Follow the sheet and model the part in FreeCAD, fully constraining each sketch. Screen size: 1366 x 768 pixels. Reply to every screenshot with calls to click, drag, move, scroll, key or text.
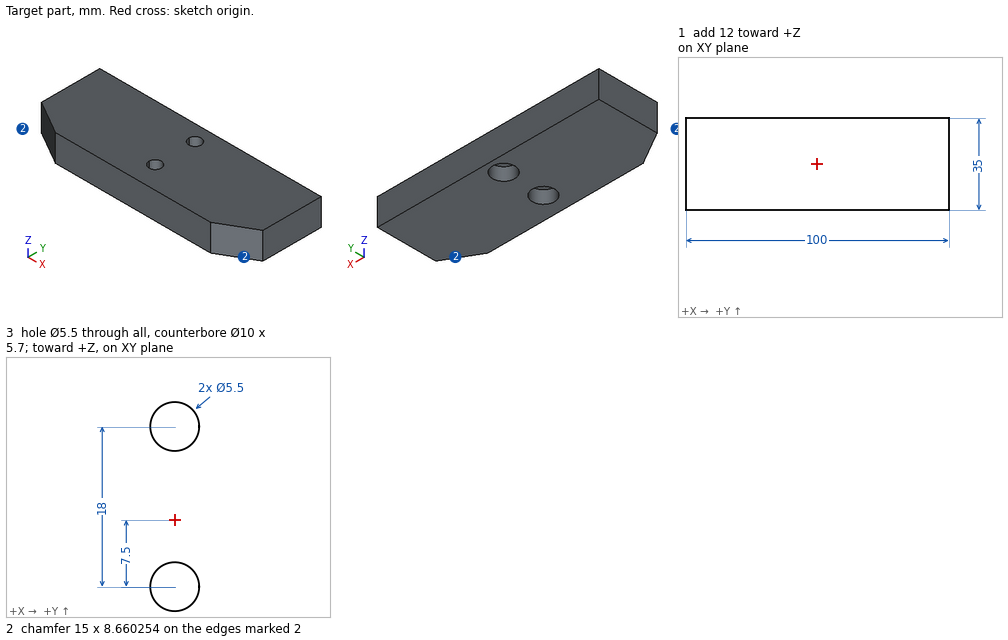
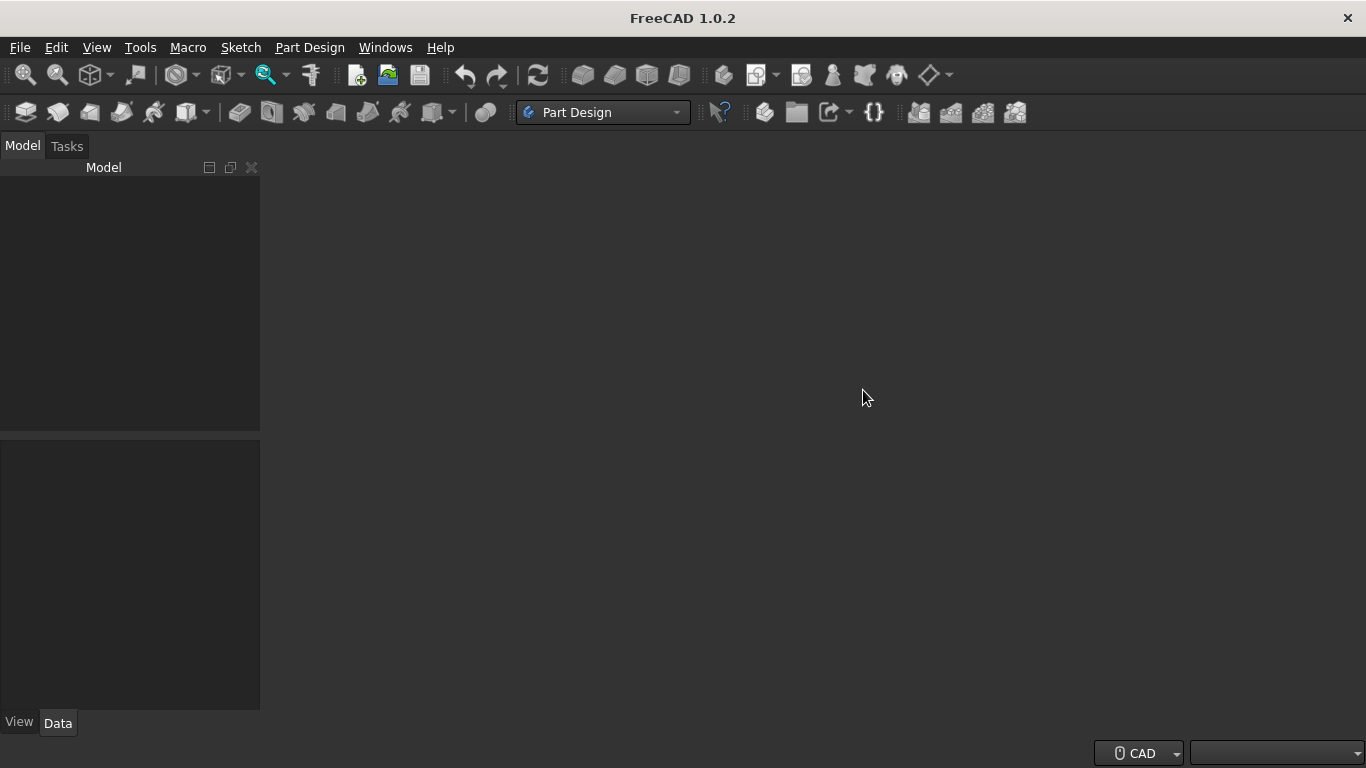
click(356, 76)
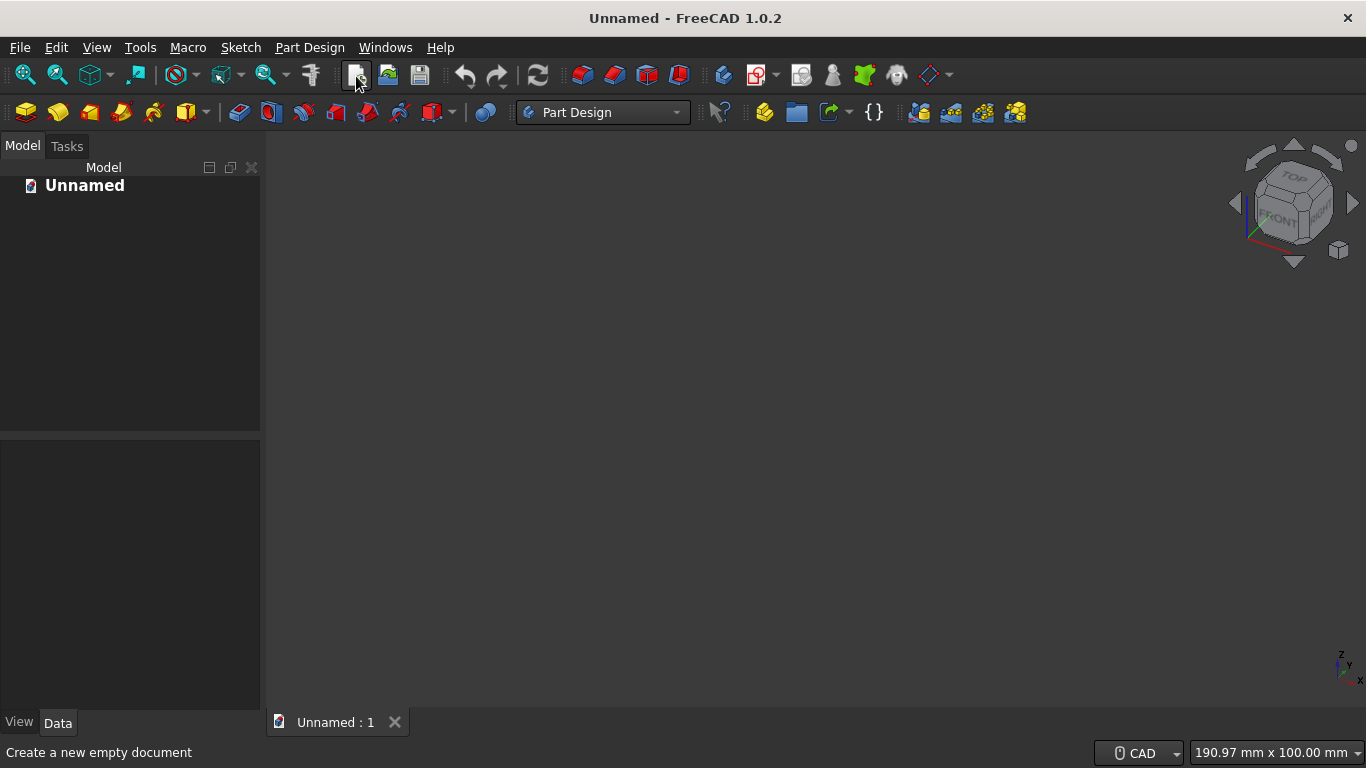
click(756, 76)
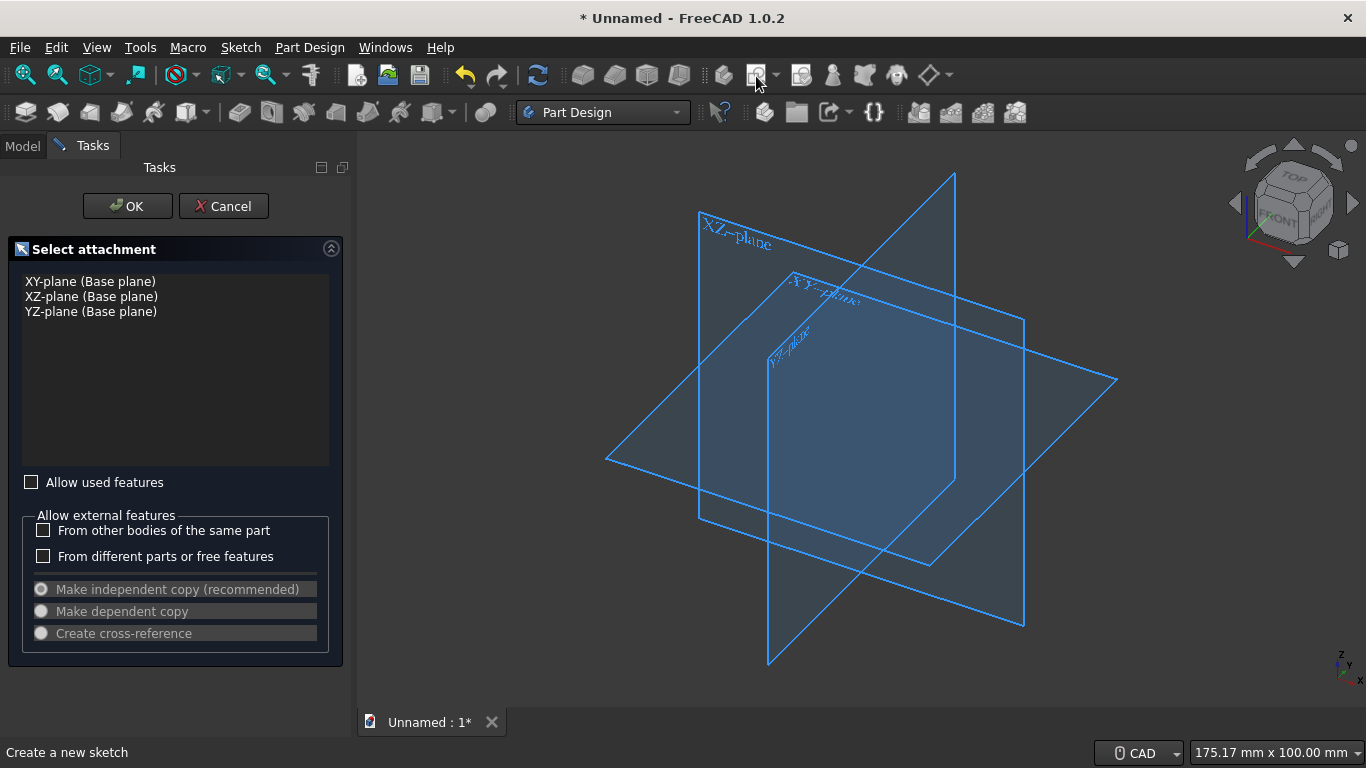
click(82, 282)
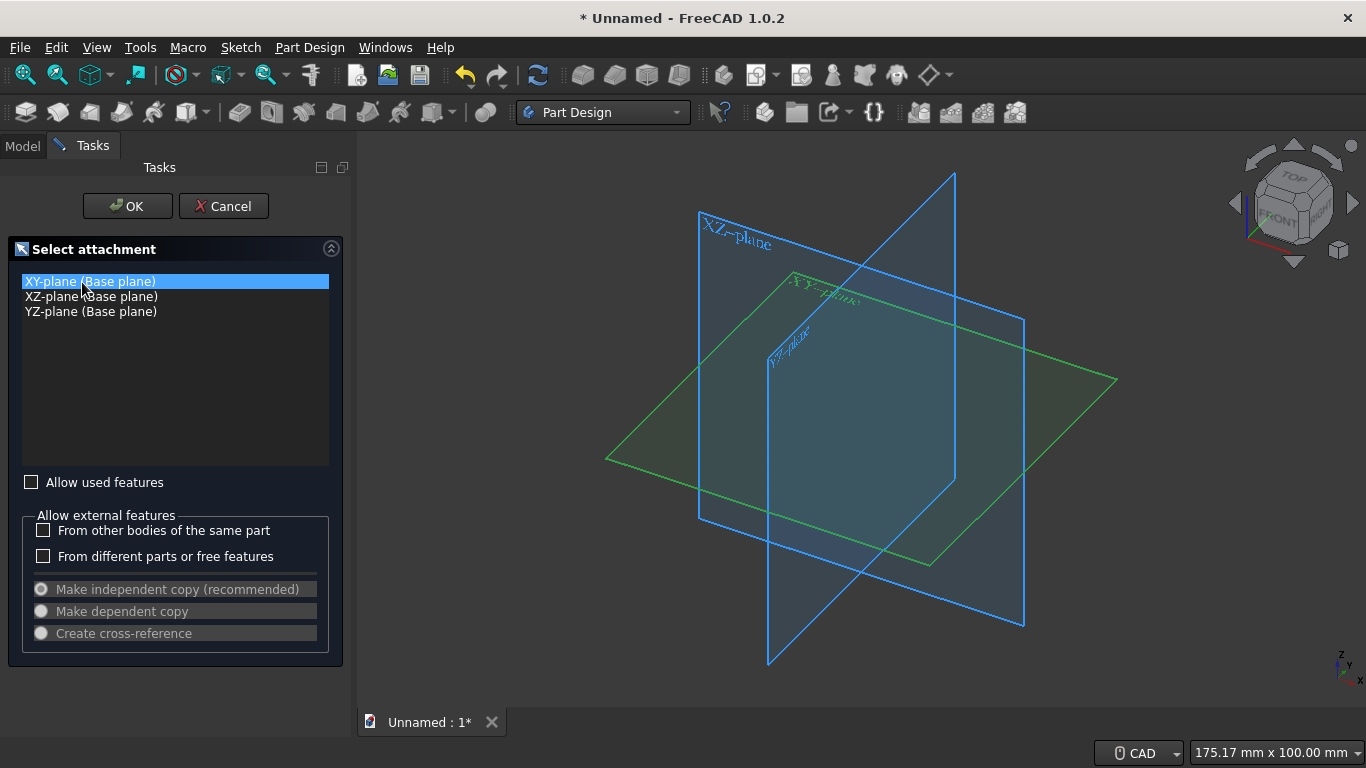
click(128, 206)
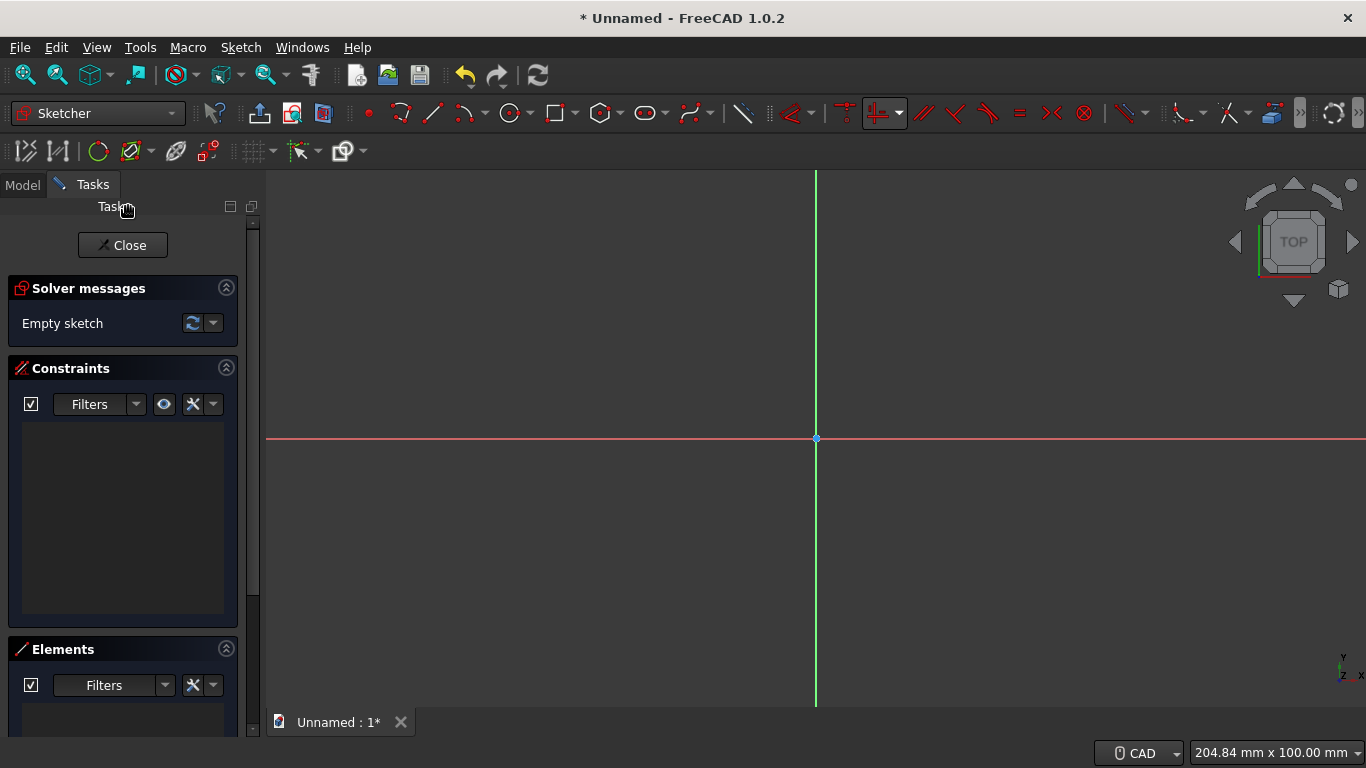
click(578, 114)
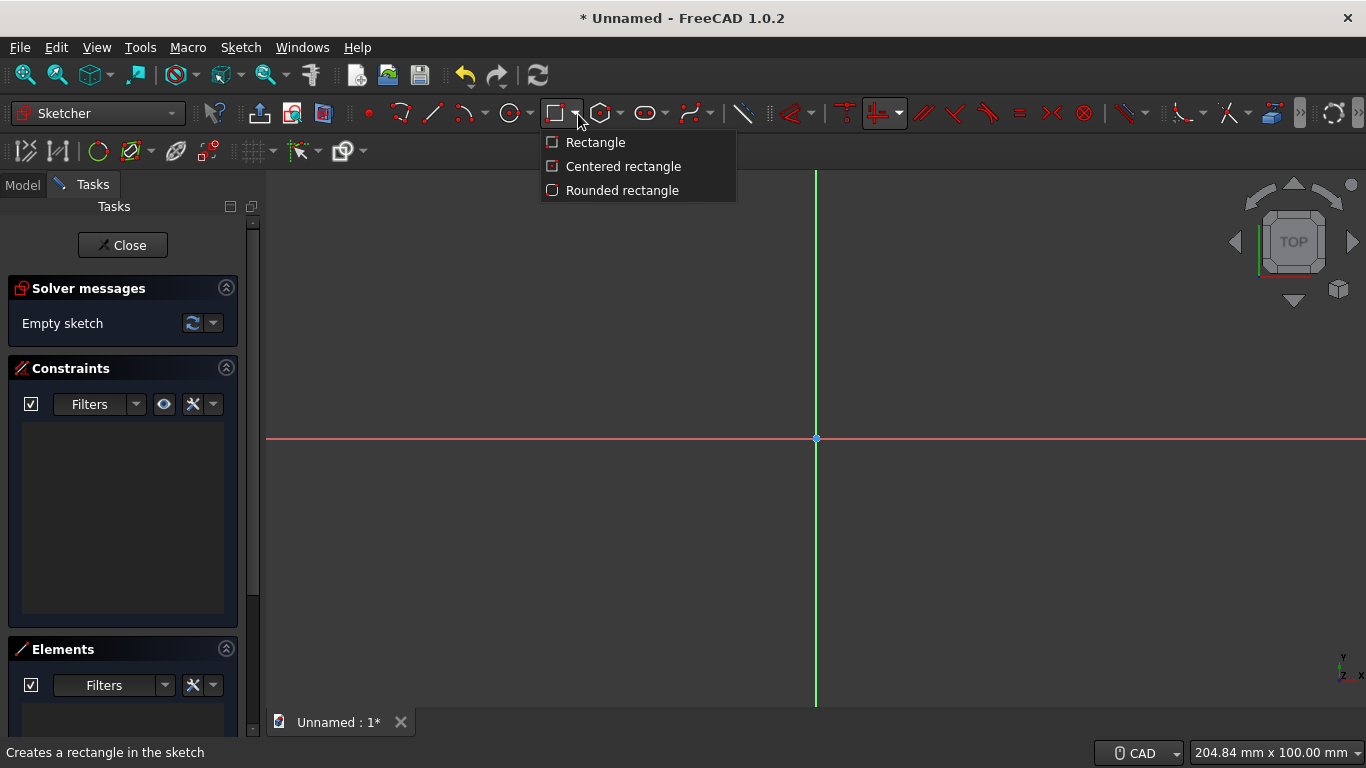
click(638, 166)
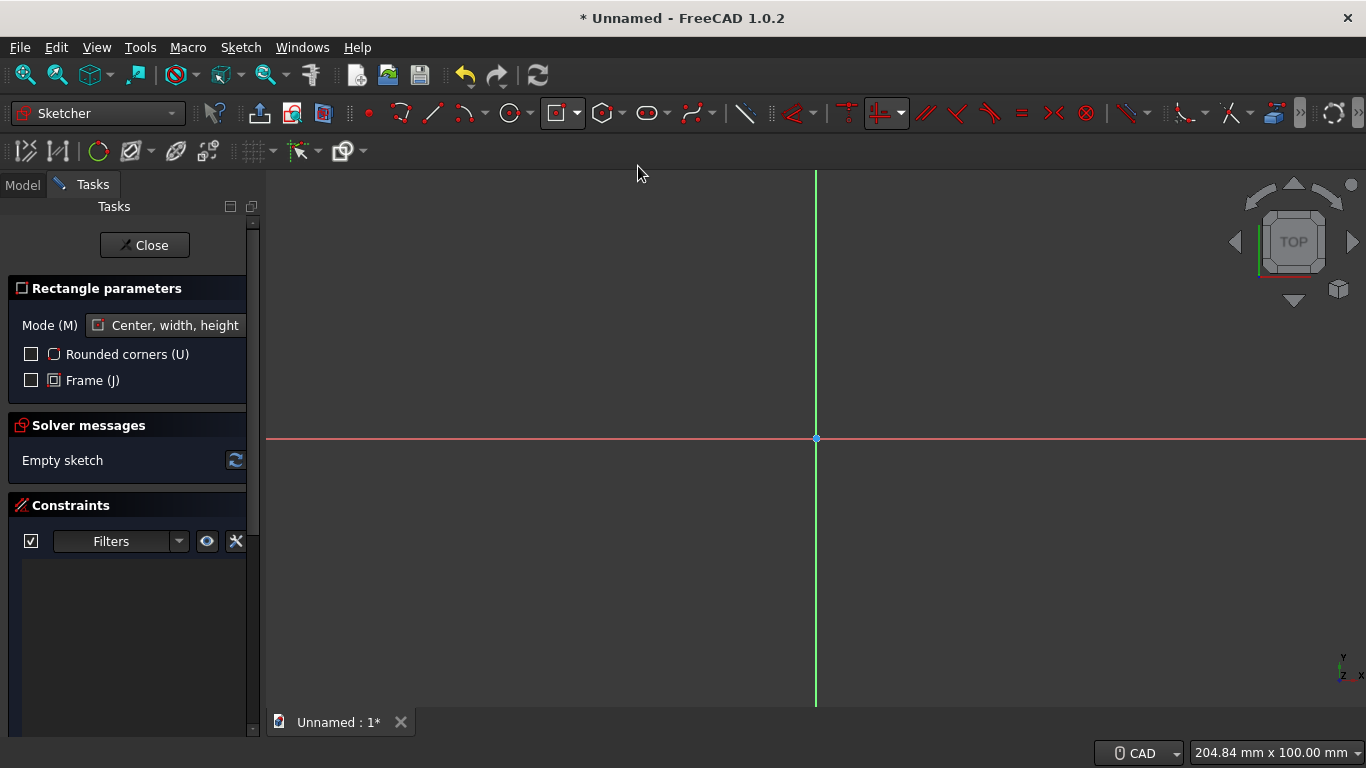
click(816, 438)
move(1084, 345)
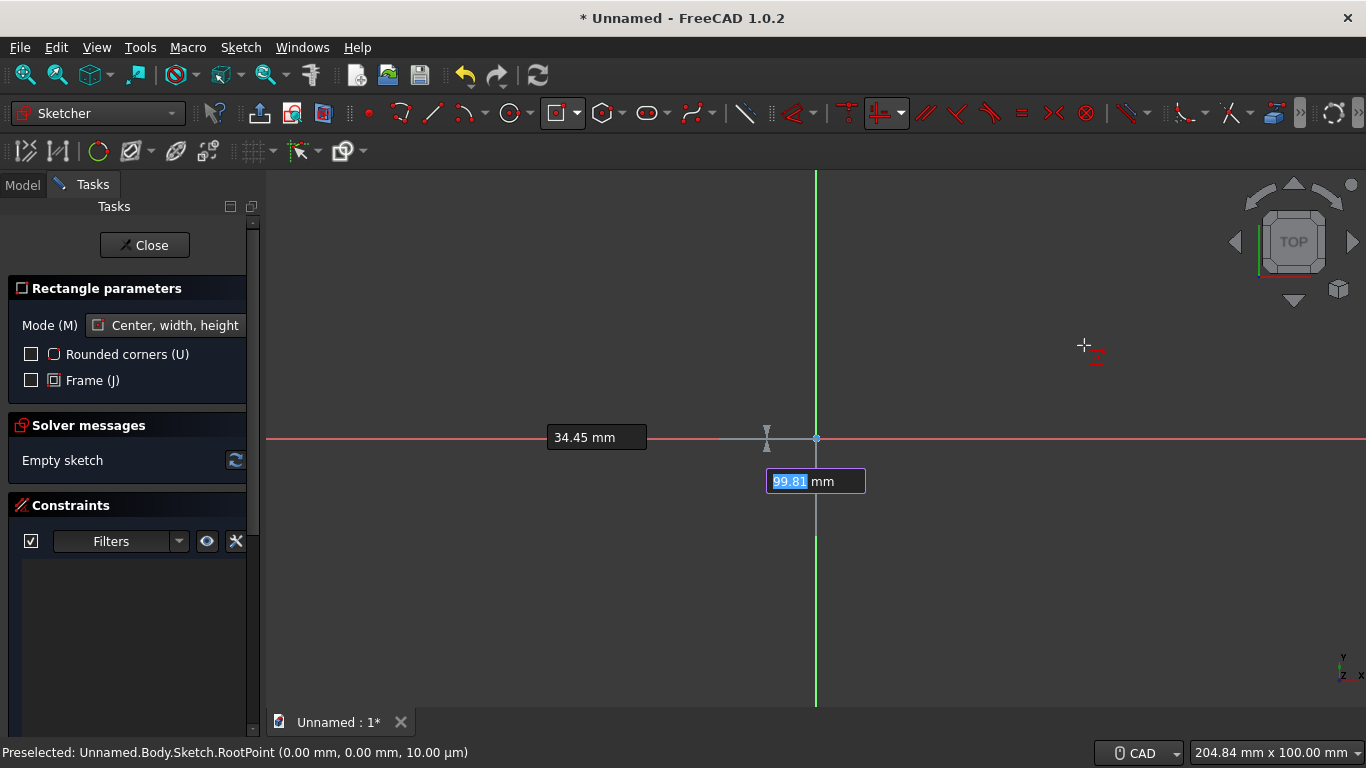
text(100)
key(Tab)
text(35)
key(Return)
key(Escape)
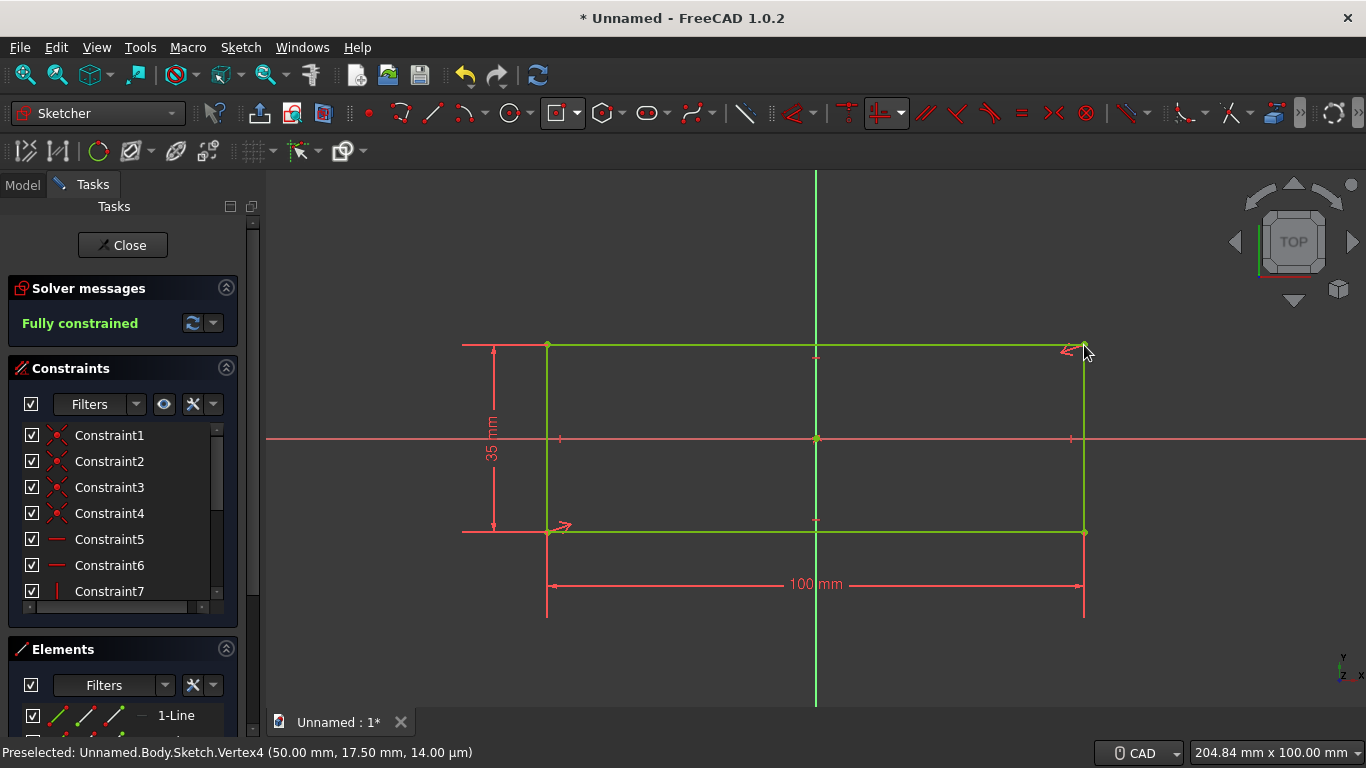
click(123, 245)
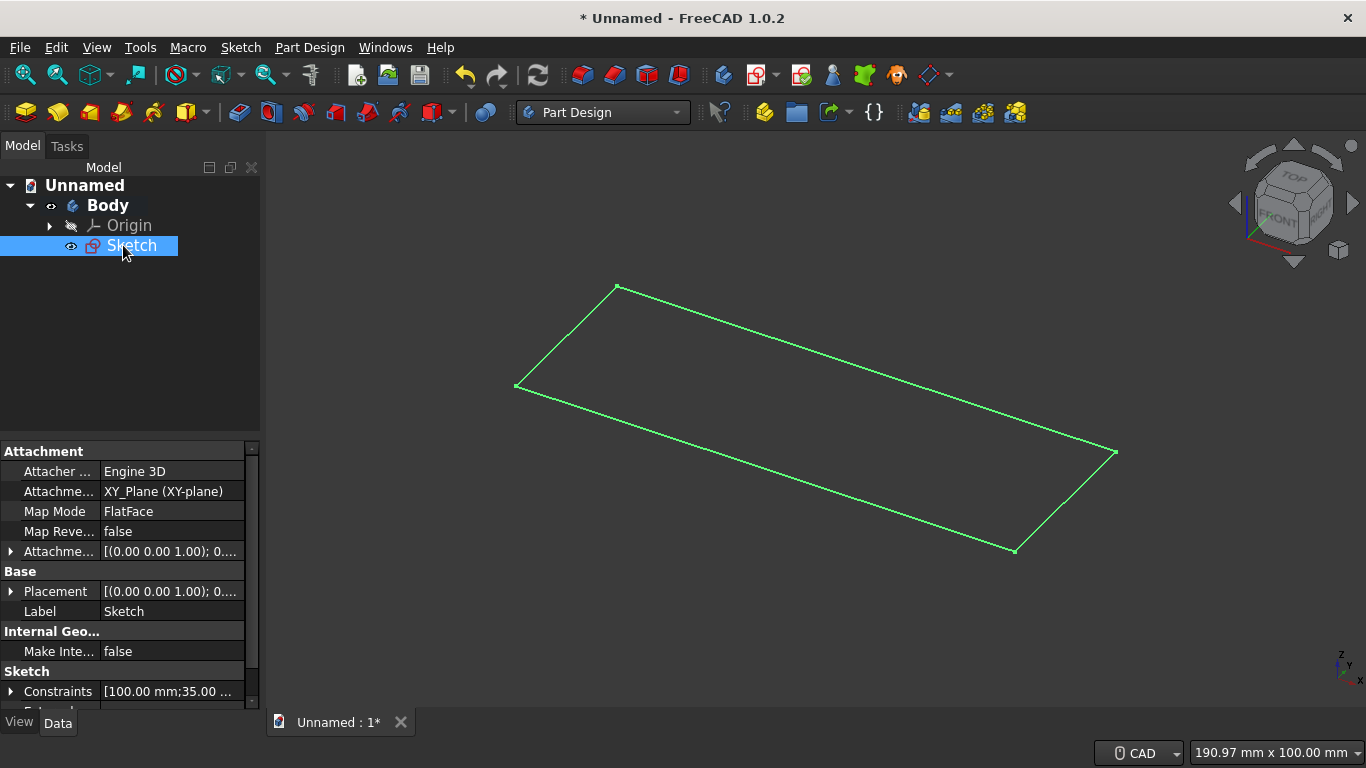
click(26, 112)